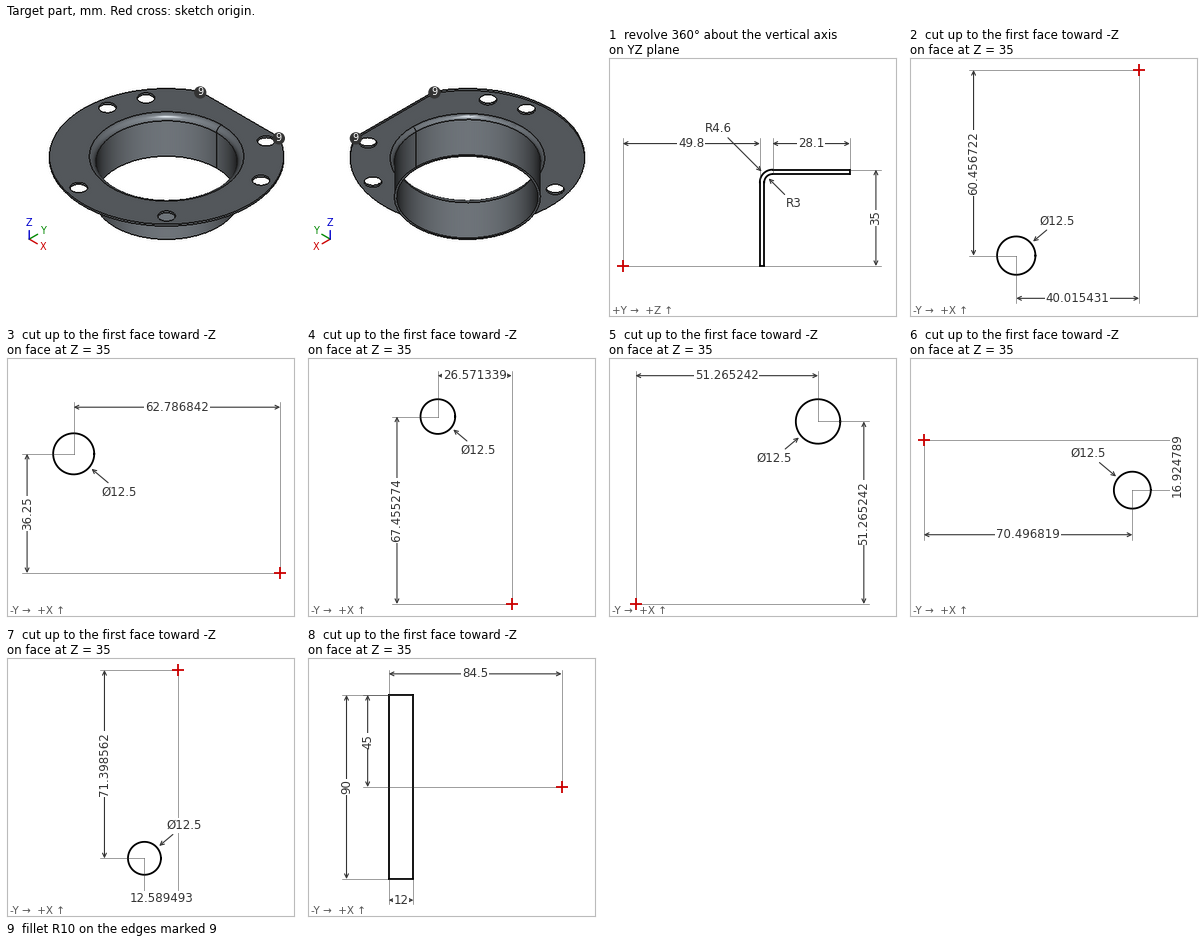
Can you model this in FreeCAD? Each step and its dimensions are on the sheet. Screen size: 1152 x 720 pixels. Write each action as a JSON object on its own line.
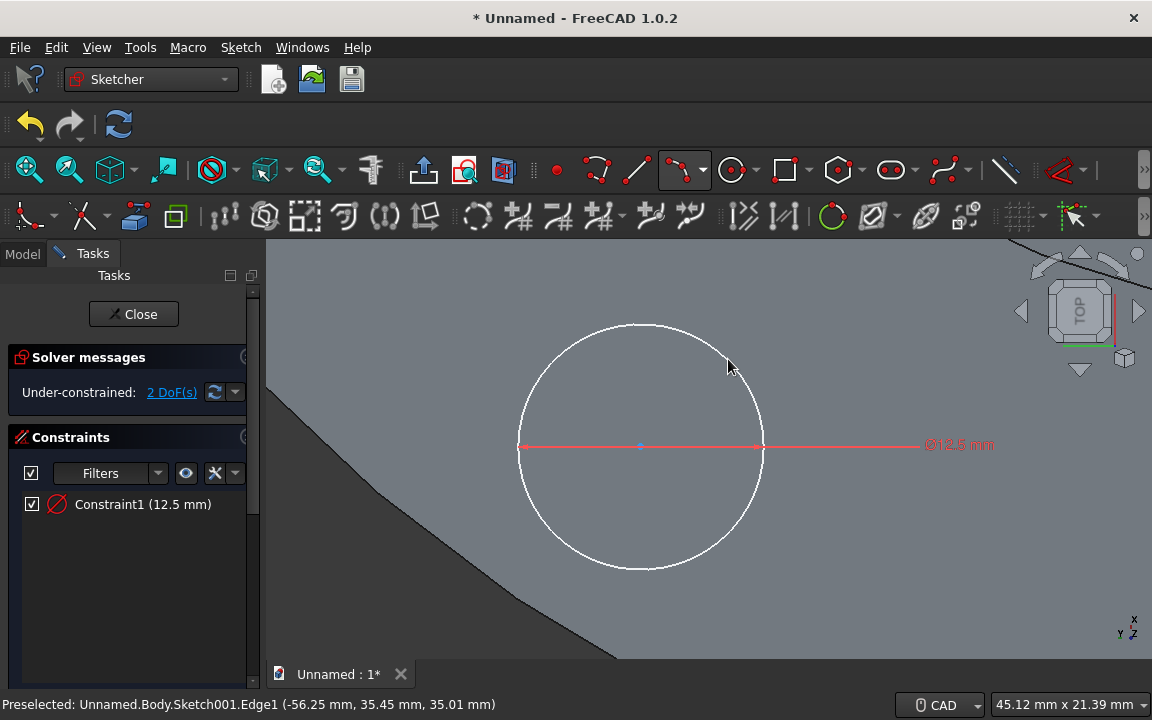
{"action": "left_click", "coordinate": [641, 447]}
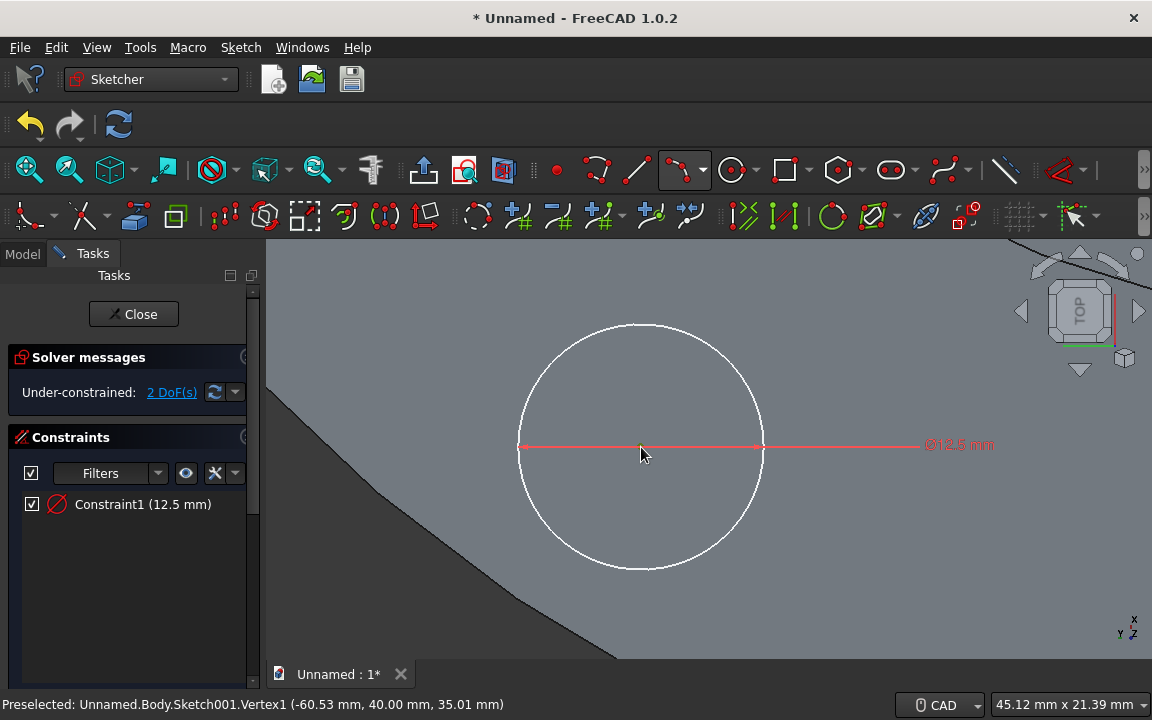
{"action": "key", "text": "l"}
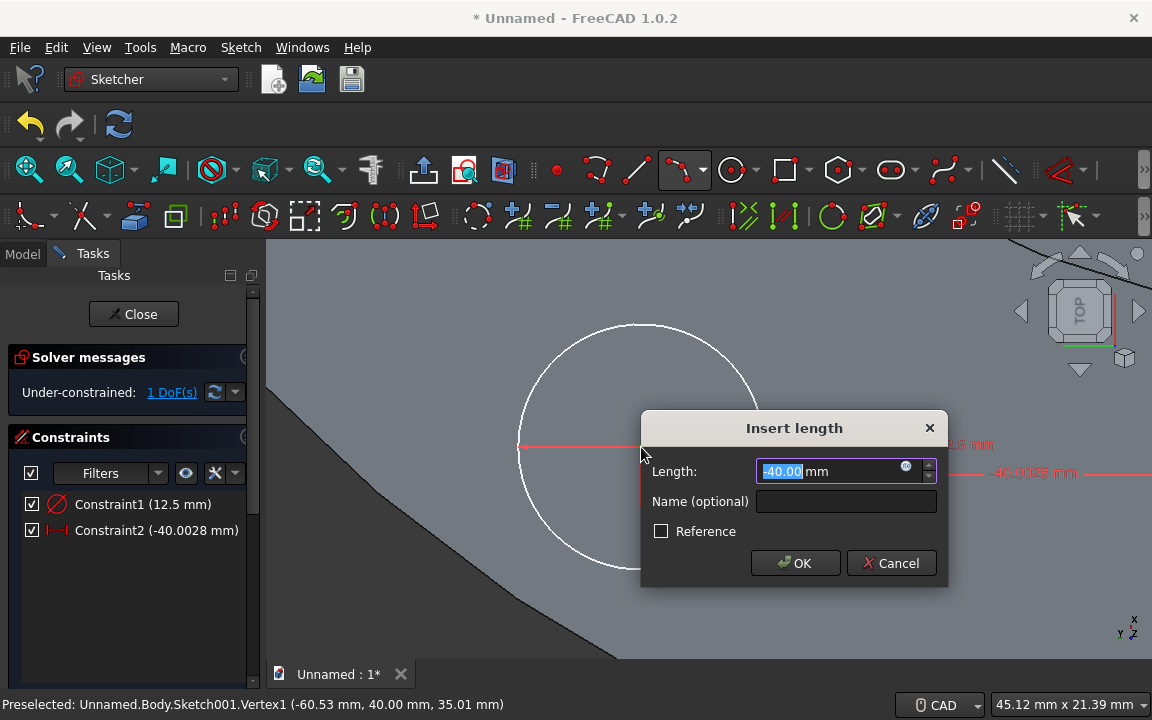
{"action": "type", "text": "-40.015431"}
{"action": "key", "text": "Return"}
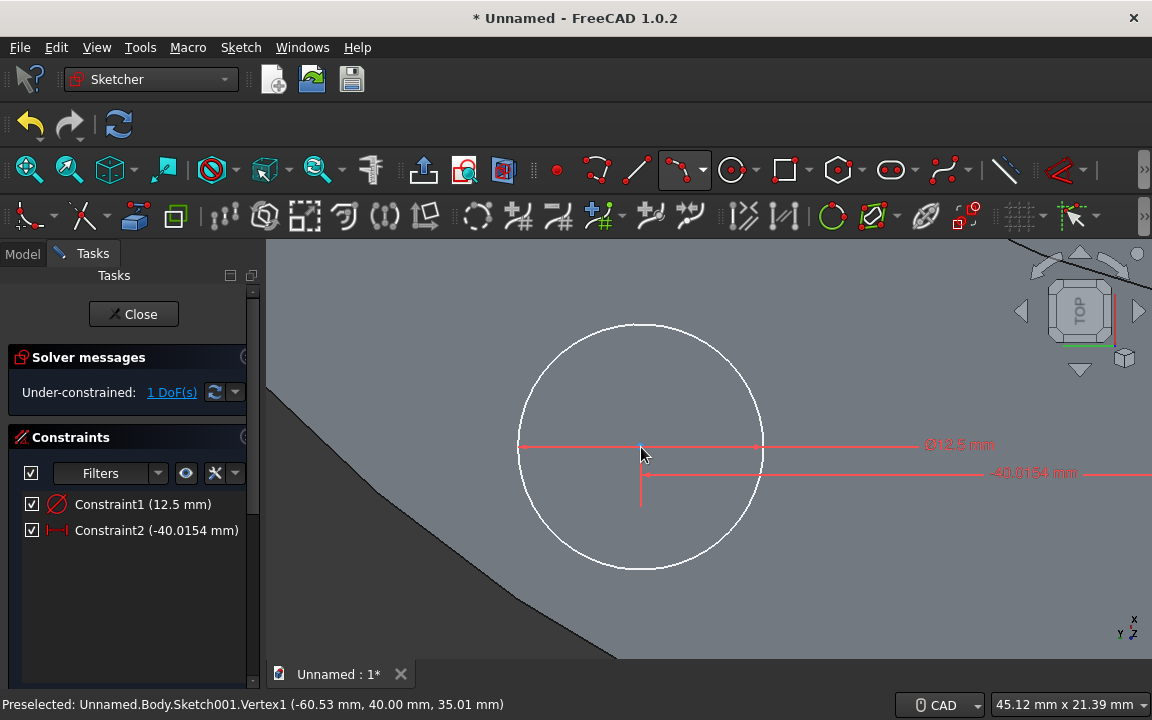
{"action": "left_click", "coordinate": [641, 447]}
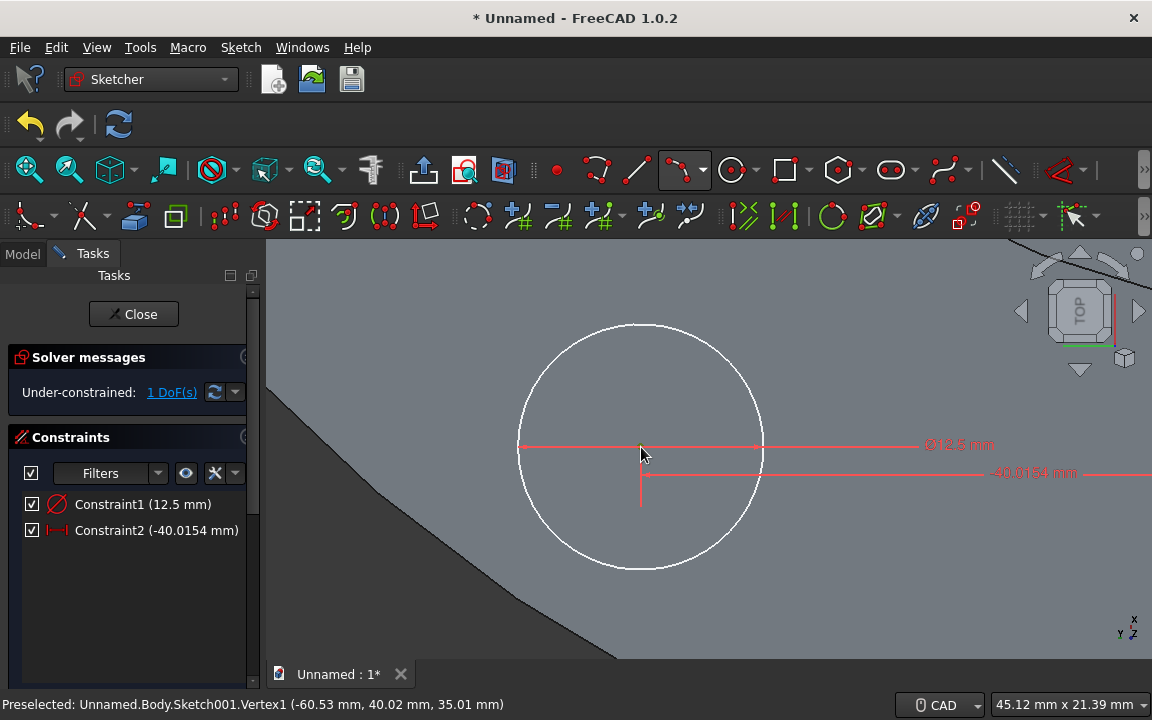
{"action": "key", "text": "i"}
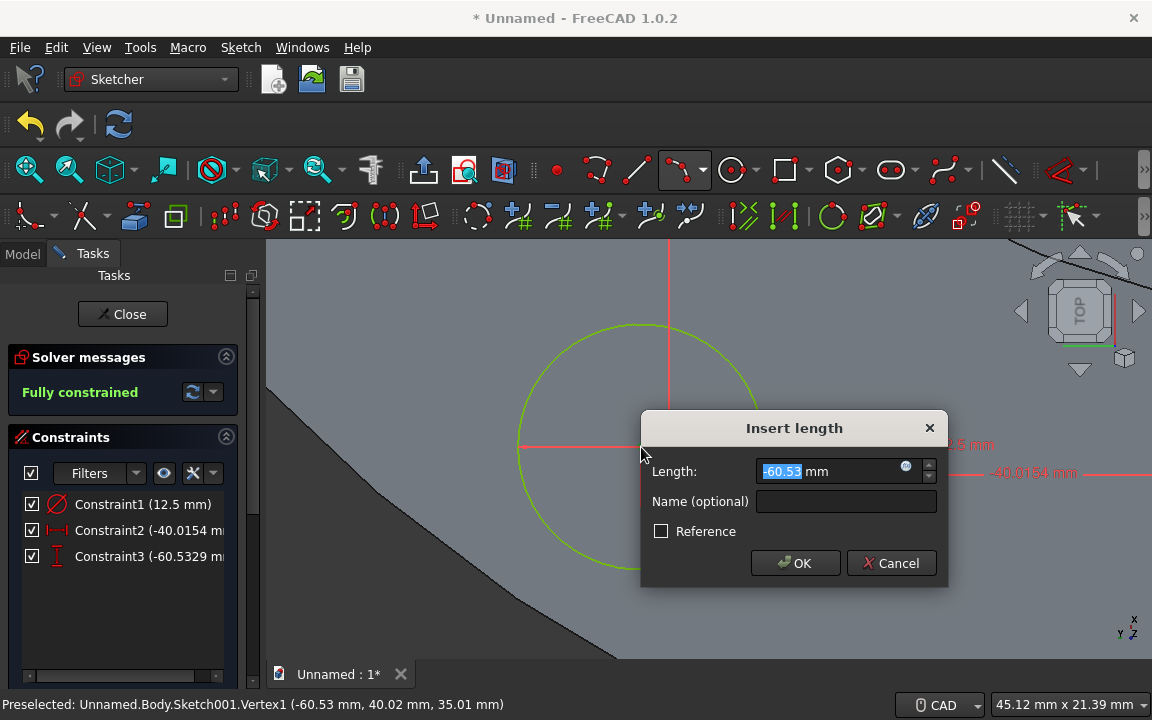
{"action": "type", "text": "-60.456722"}
{"action": "key", "text": "Return"}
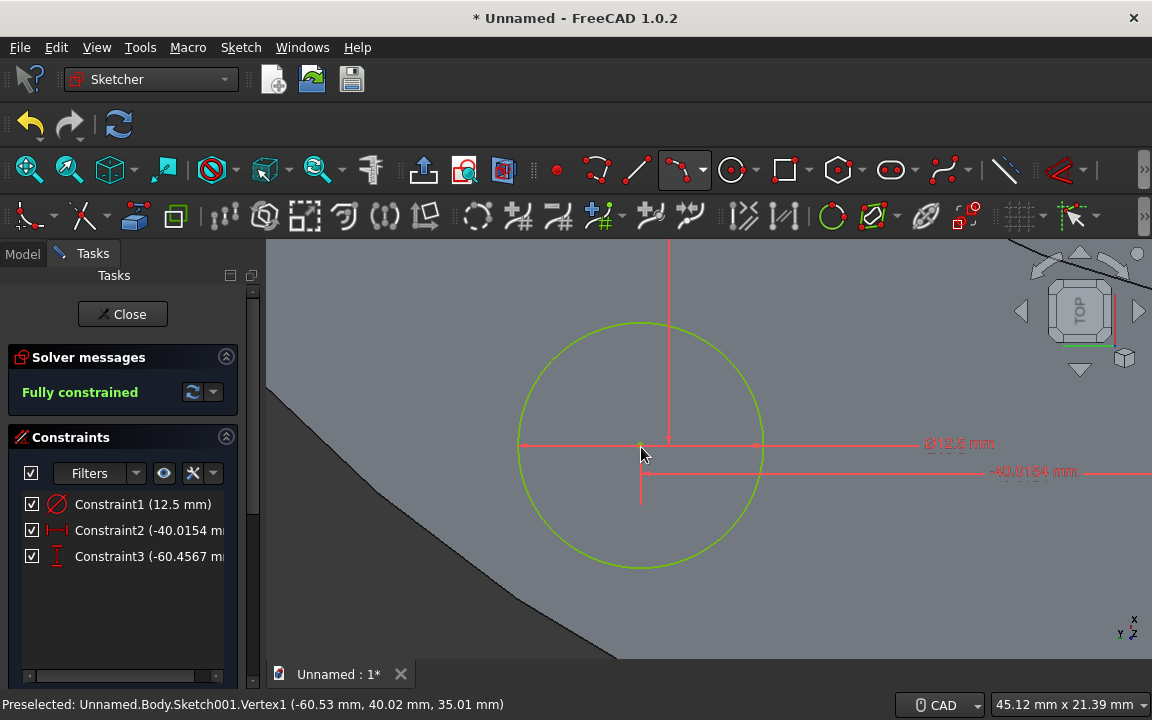
{"action": "left_click", "coordinate": [123, 314]}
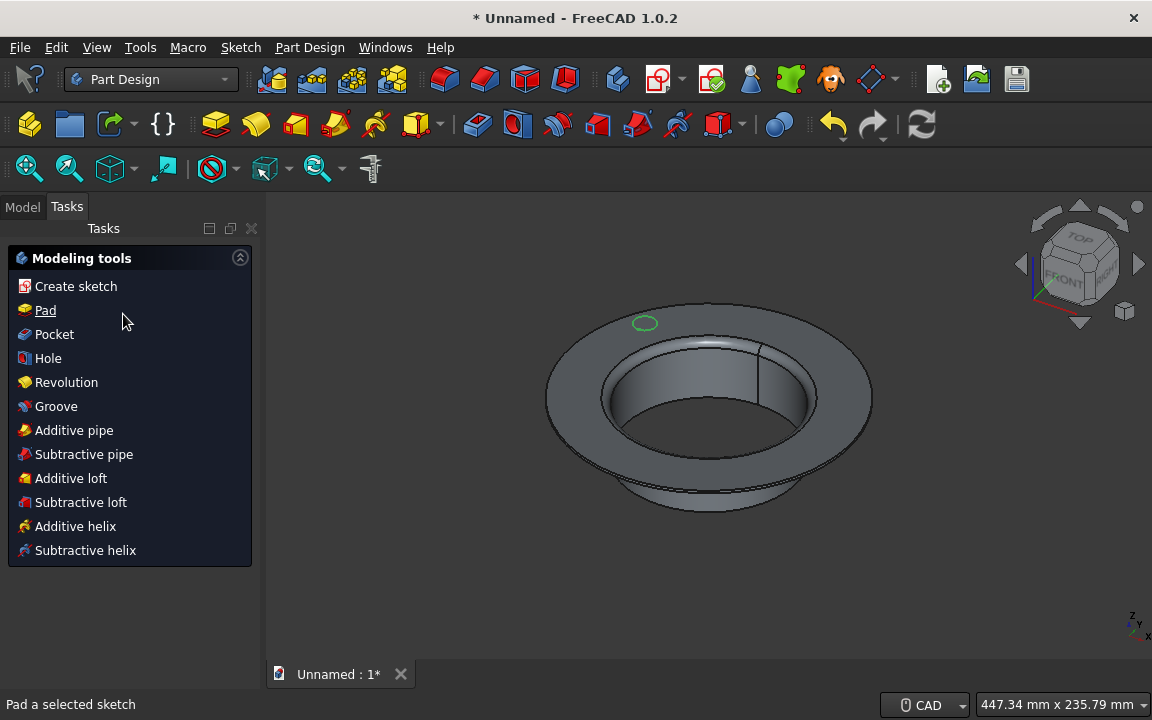
{"action": "left_click", "coordinate": [478, 124]}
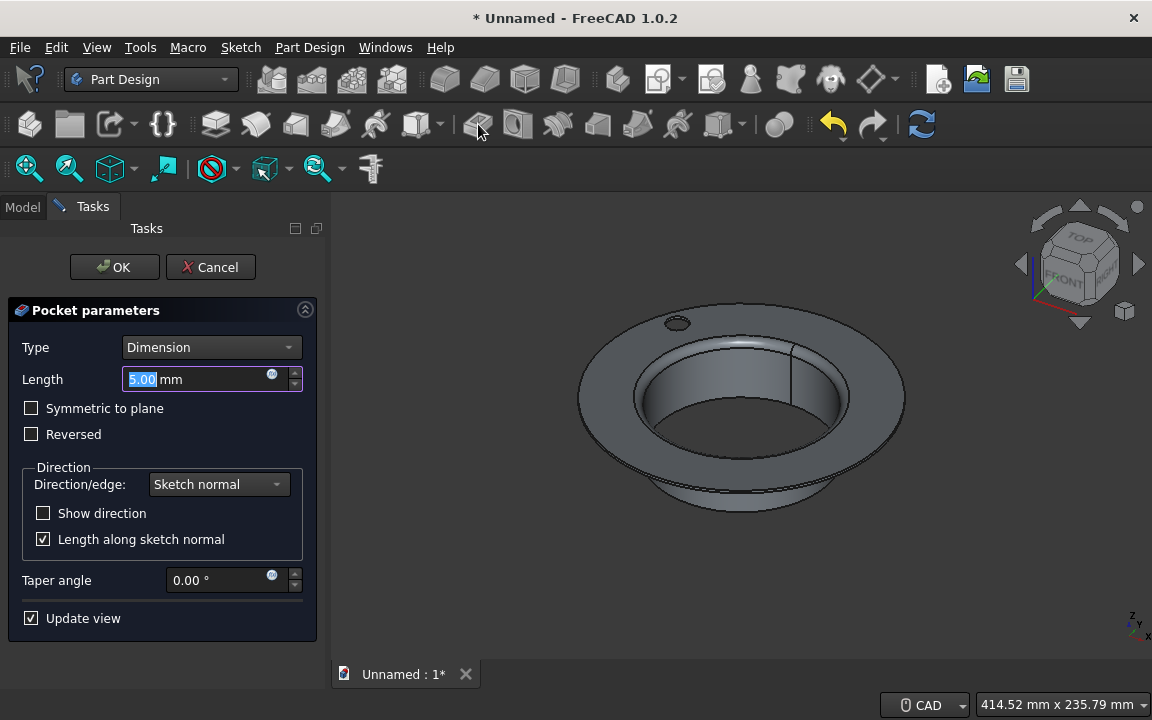
{"action": "left_click", "coordinate": [212, 348]}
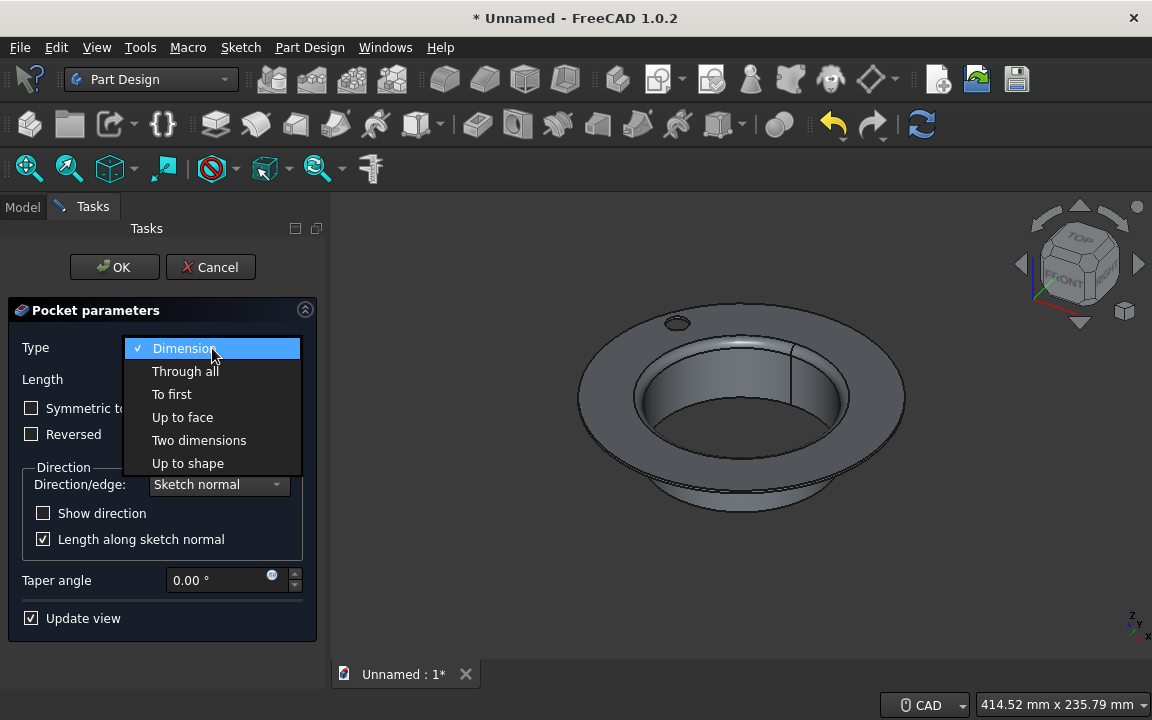
{"action": "left_click", "coordinate": [212, 394]}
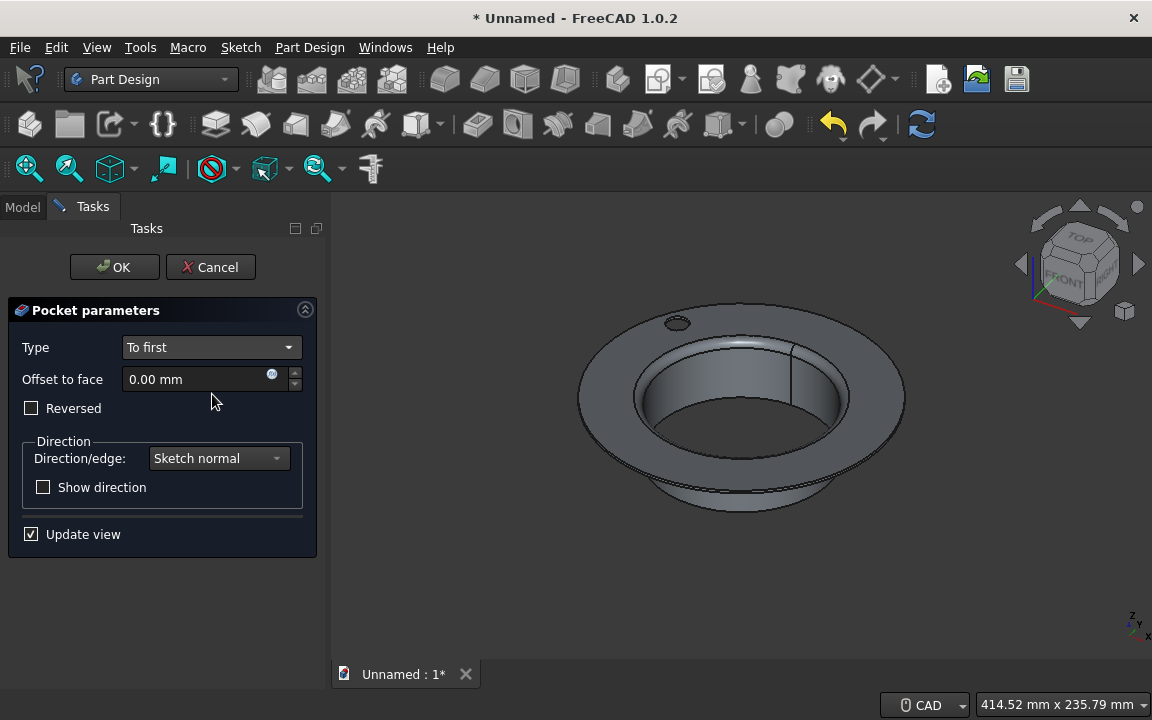
{"action": "left_click", "coordinate": [115, 267]}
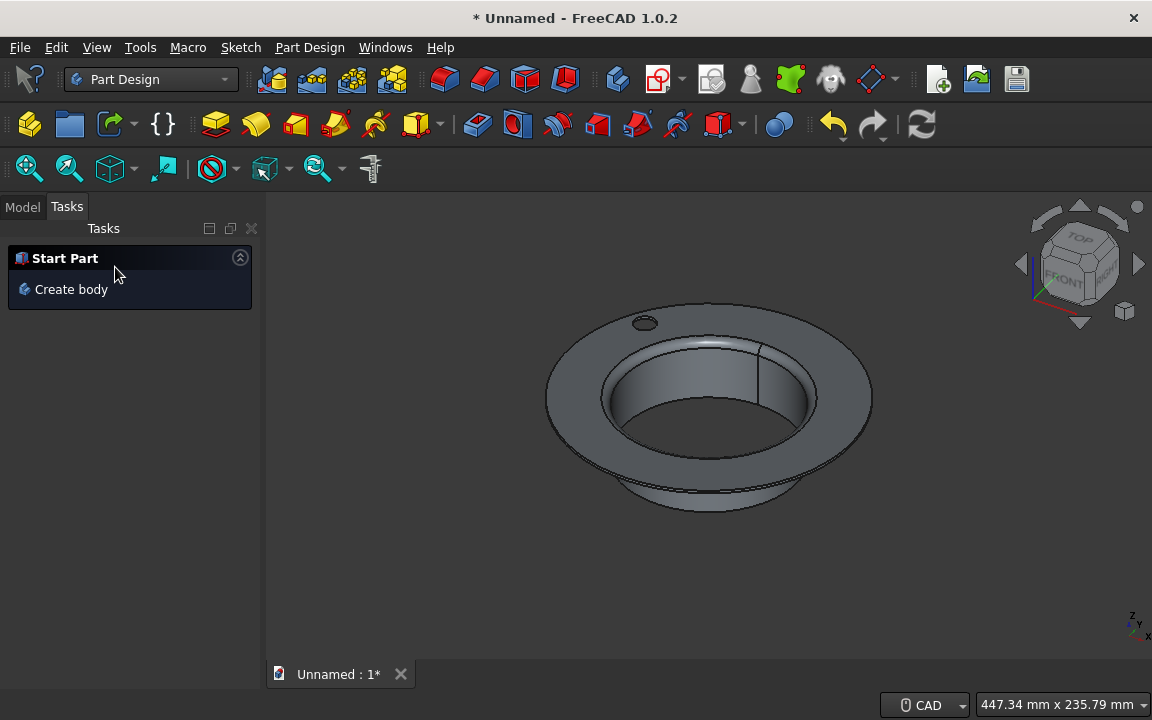
{"action": "left_click", "coordinate": [837, 377]}